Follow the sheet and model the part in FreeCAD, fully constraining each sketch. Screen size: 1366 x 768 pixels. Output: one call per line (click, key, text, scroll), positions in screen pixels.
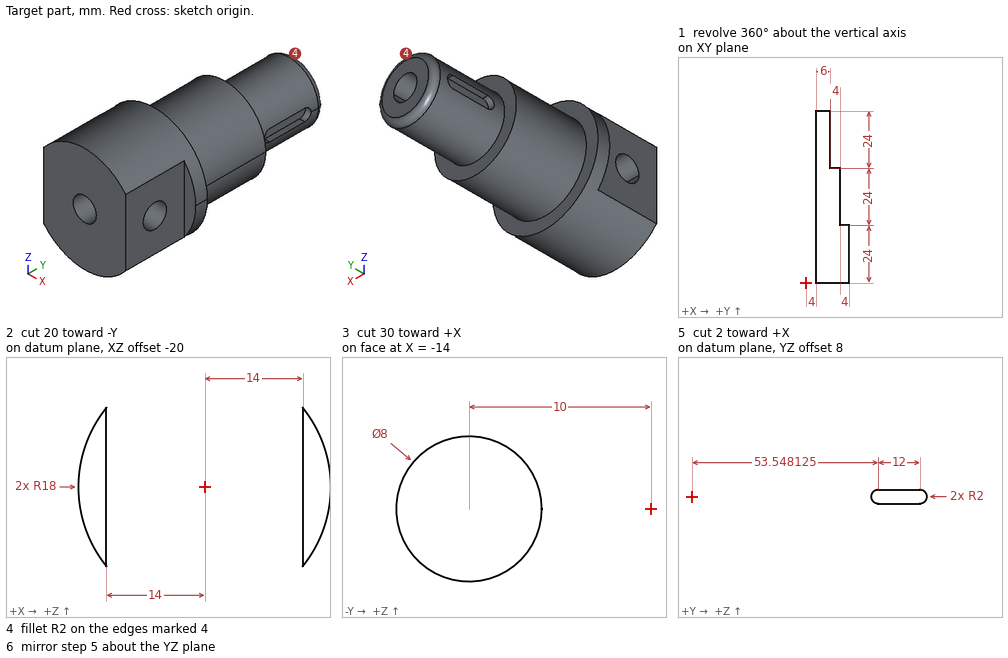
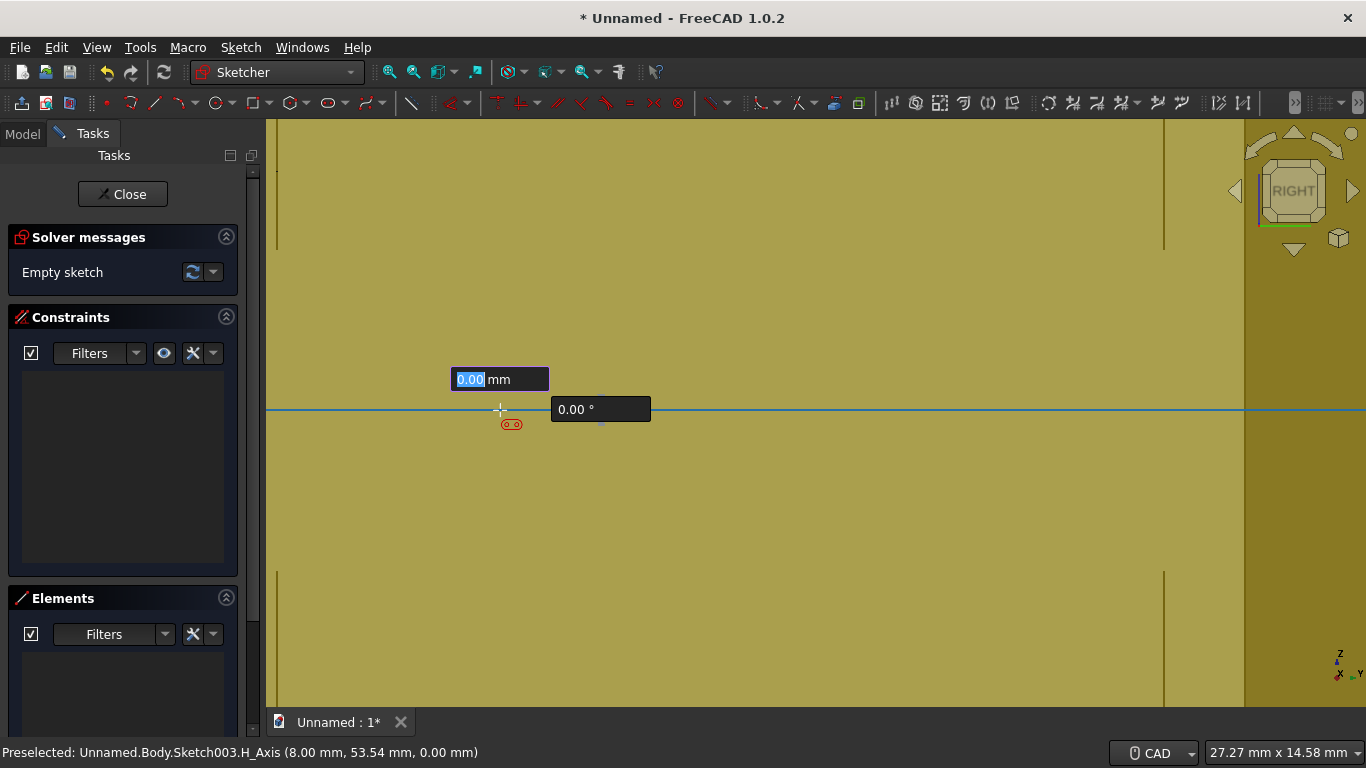
click(984, 401)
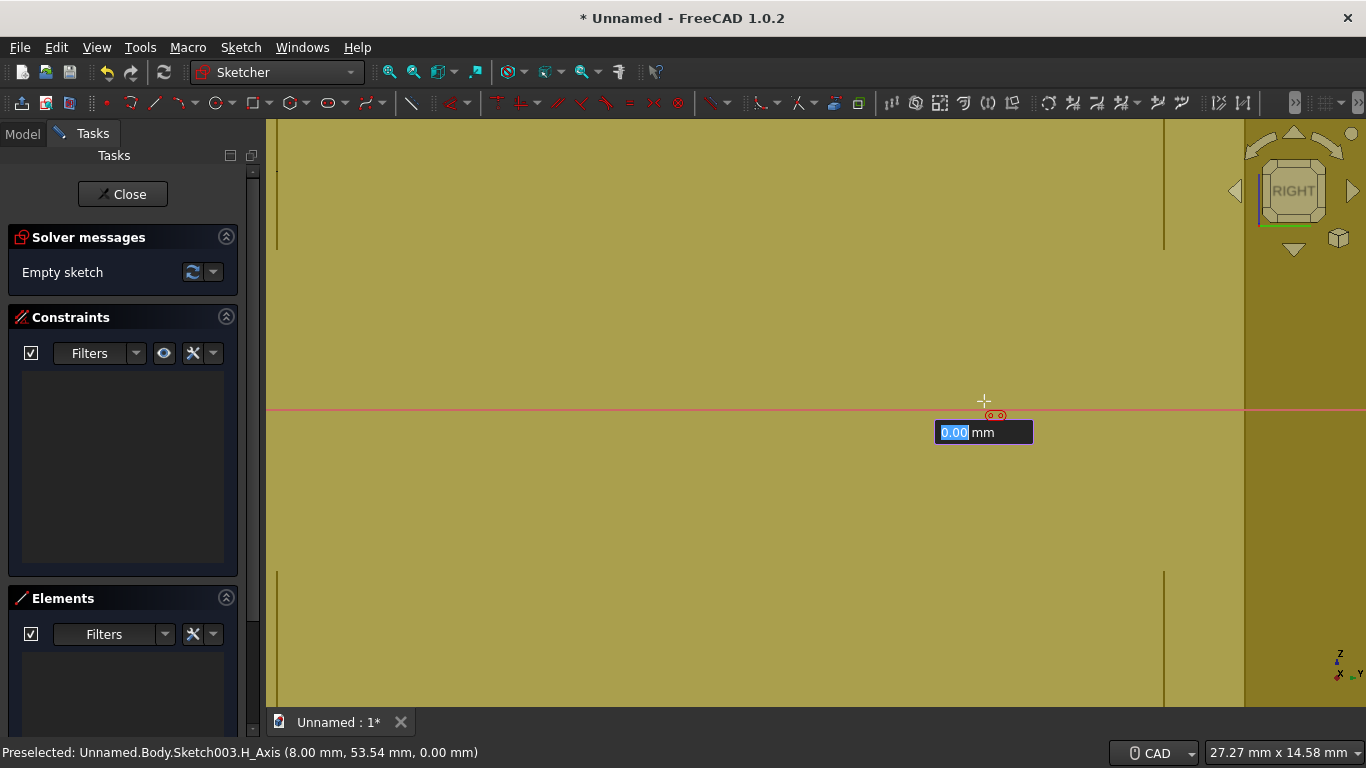
click(742, 491)
key(Escape)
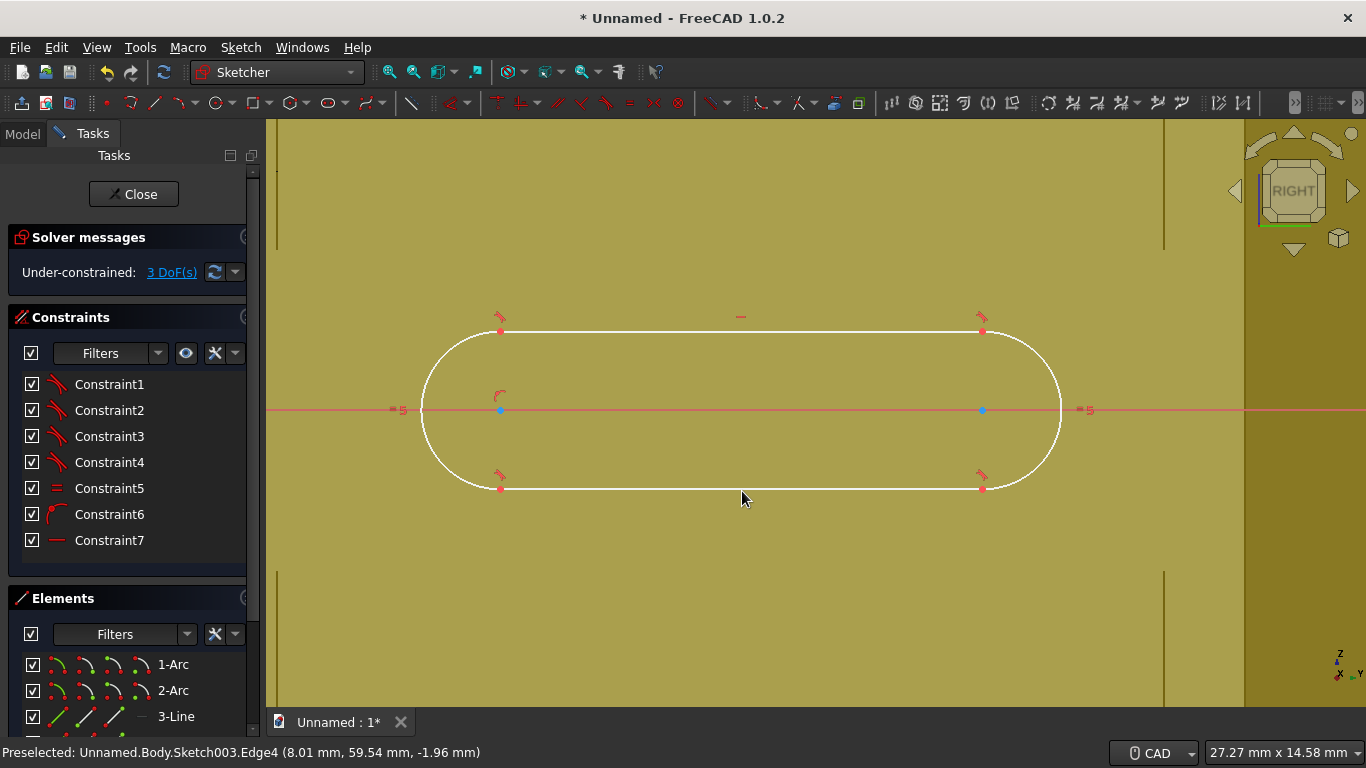
click(450, 104)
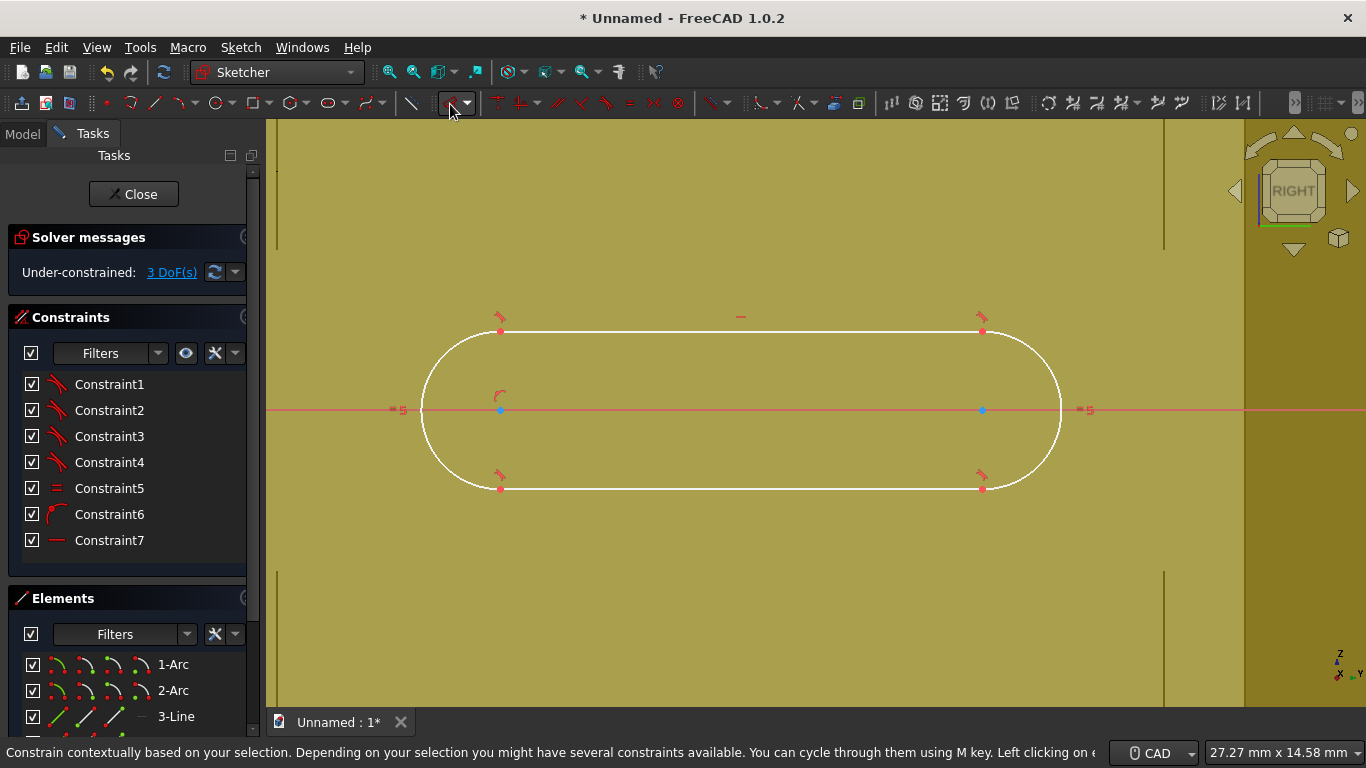
click(436, 364)
click(410, 345)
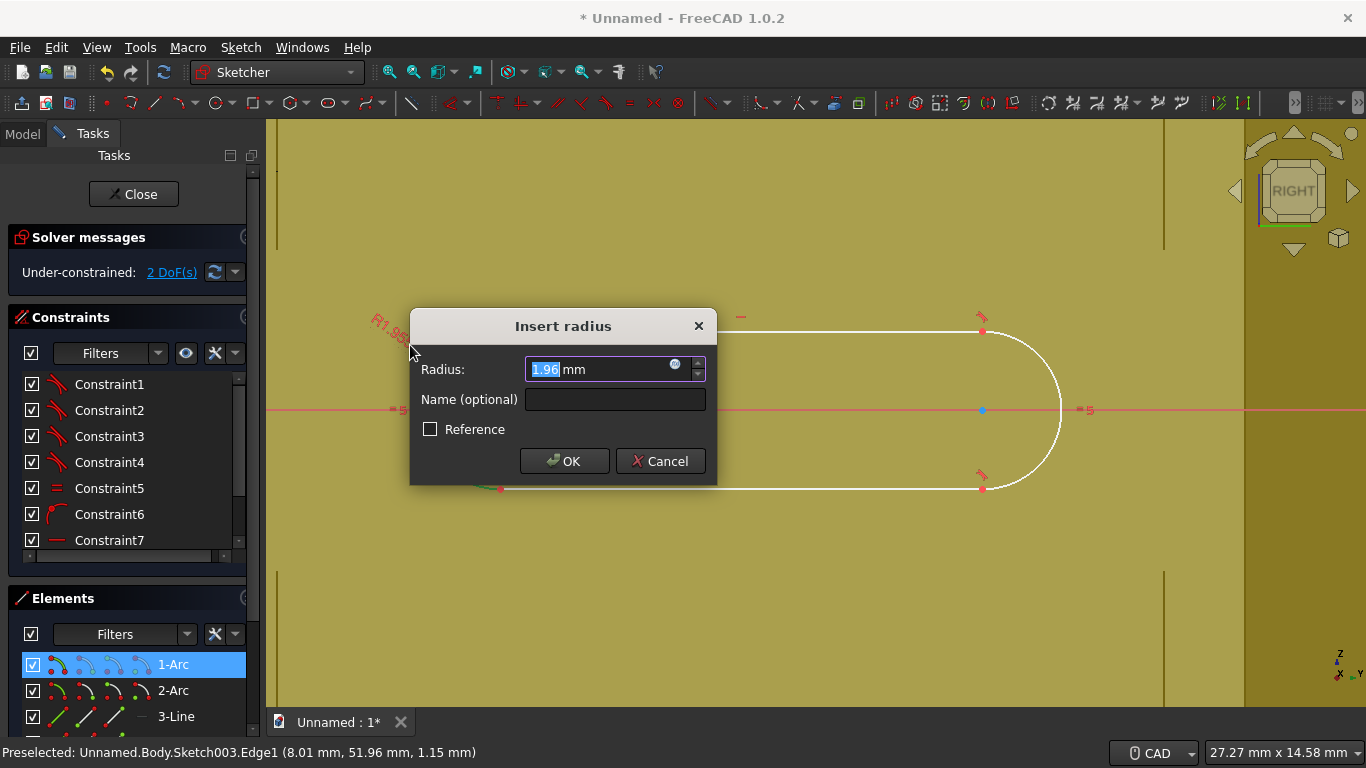
text(2)
key(Return)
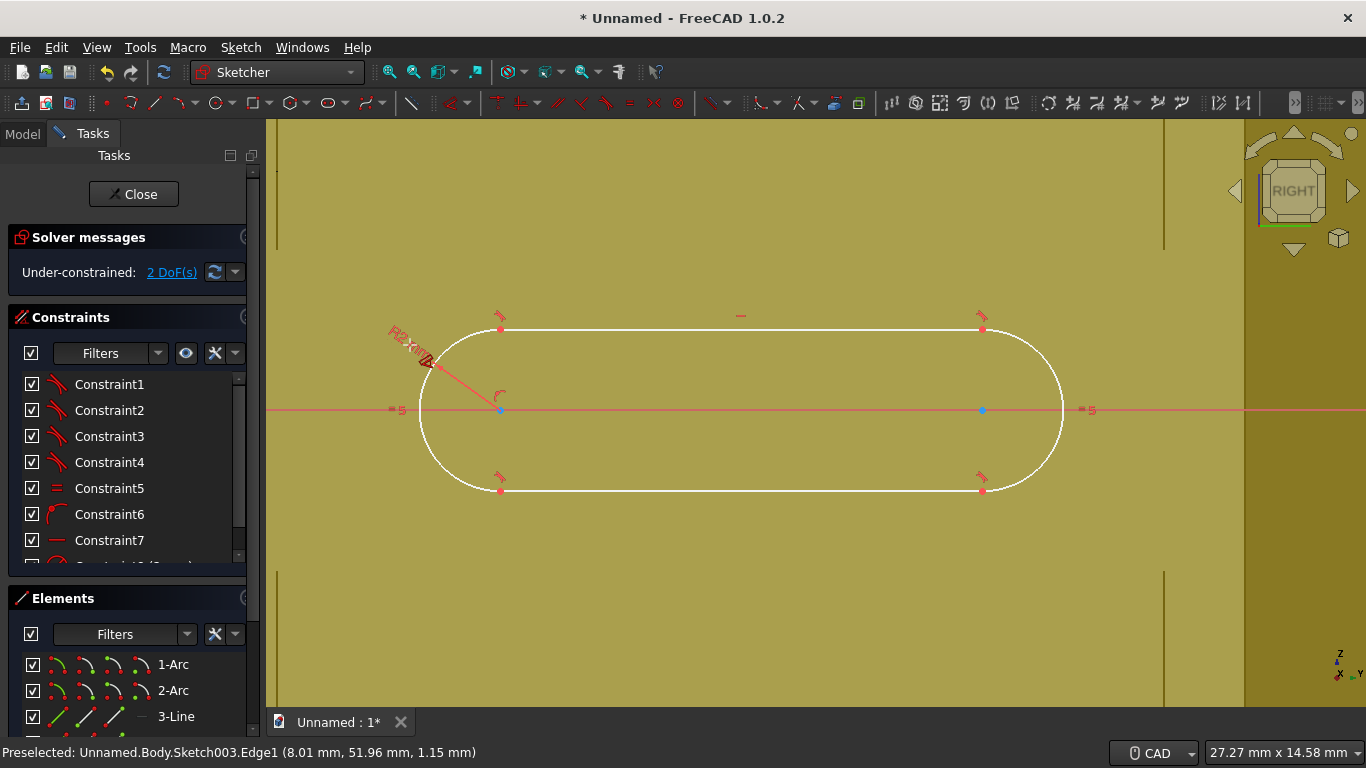
click(645, 330)
click(741, 296)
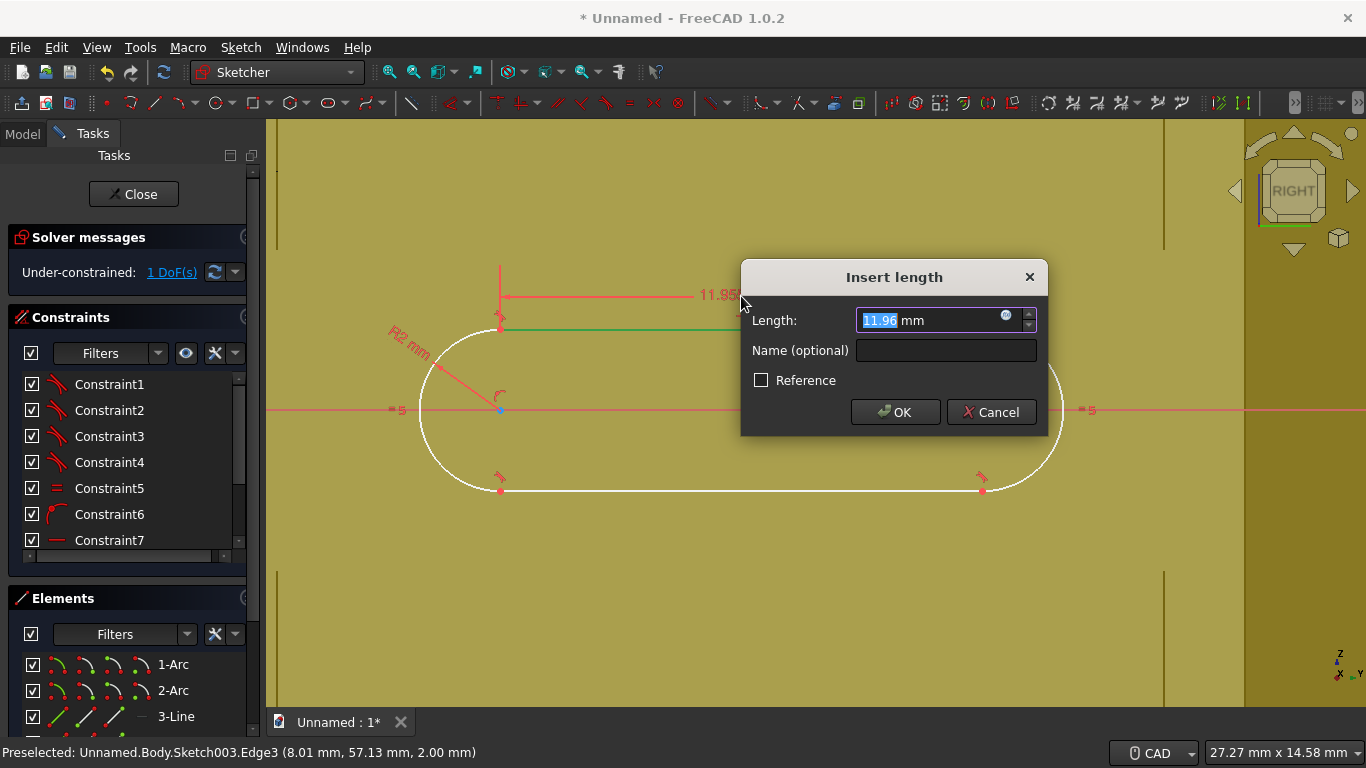
text(12)
key(Return)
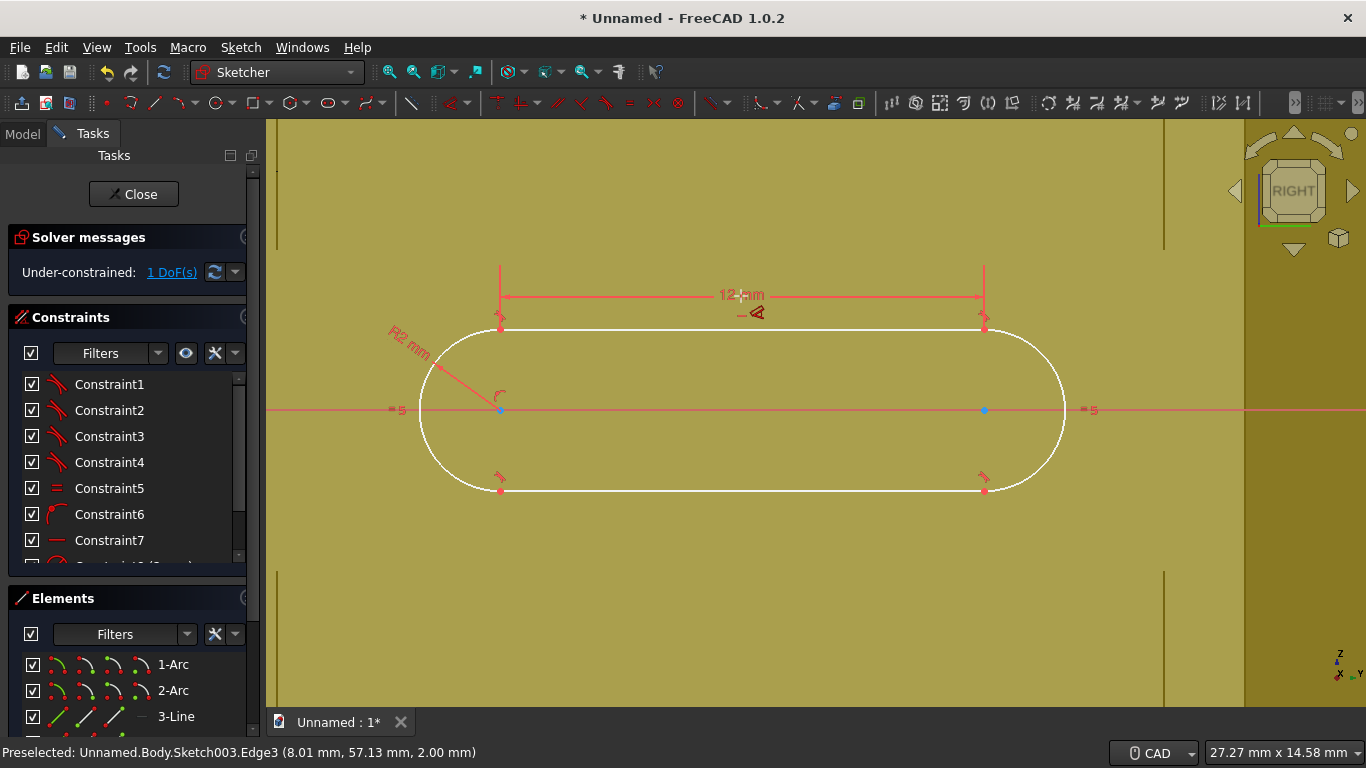
click(500, 330)
click(397, 296)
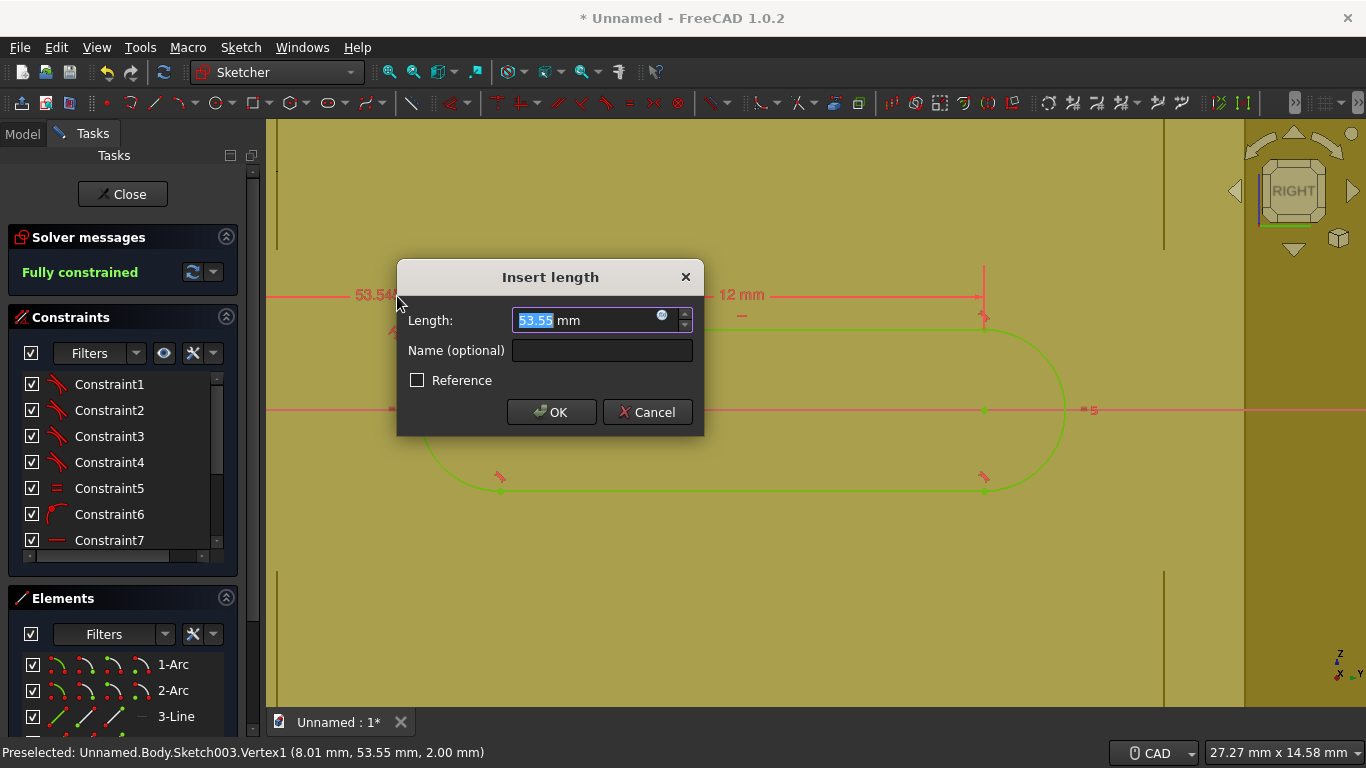
text(53.548125)
key(Return)
key(Escape)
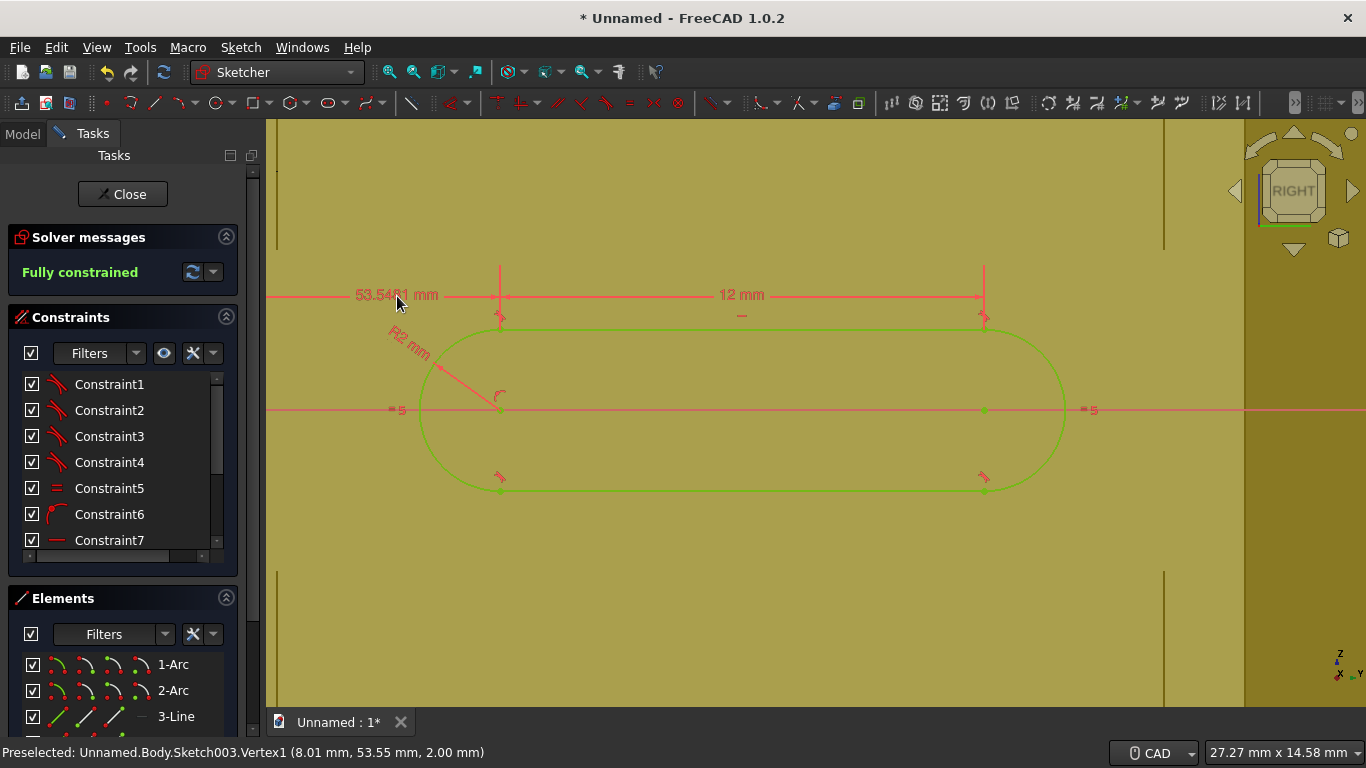
click(123, 194)